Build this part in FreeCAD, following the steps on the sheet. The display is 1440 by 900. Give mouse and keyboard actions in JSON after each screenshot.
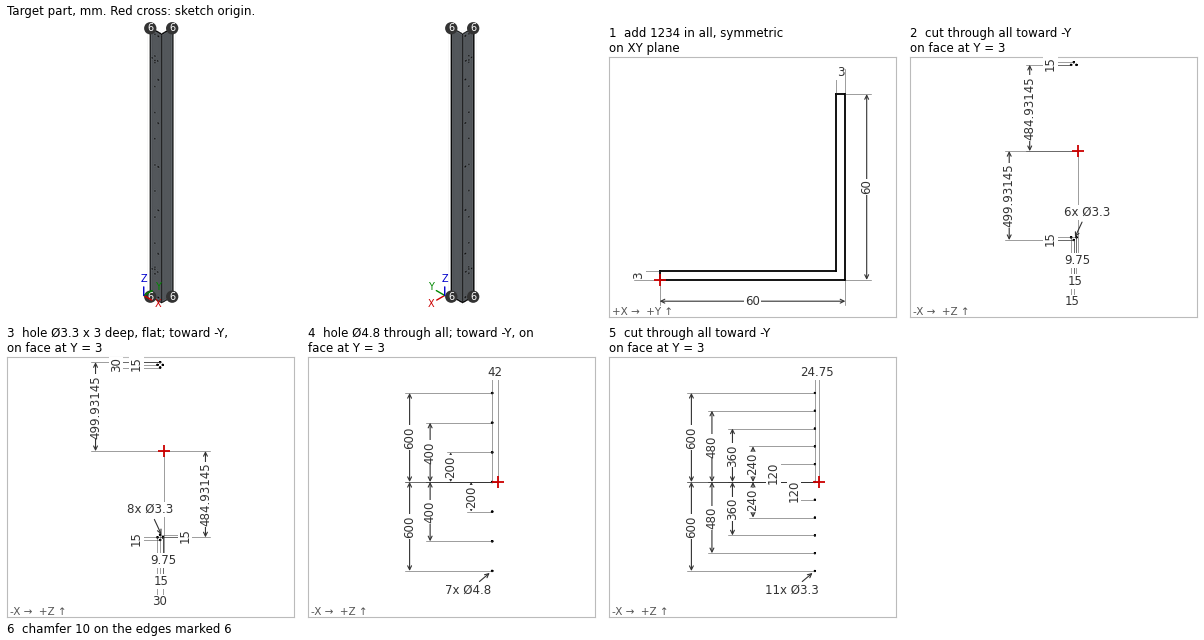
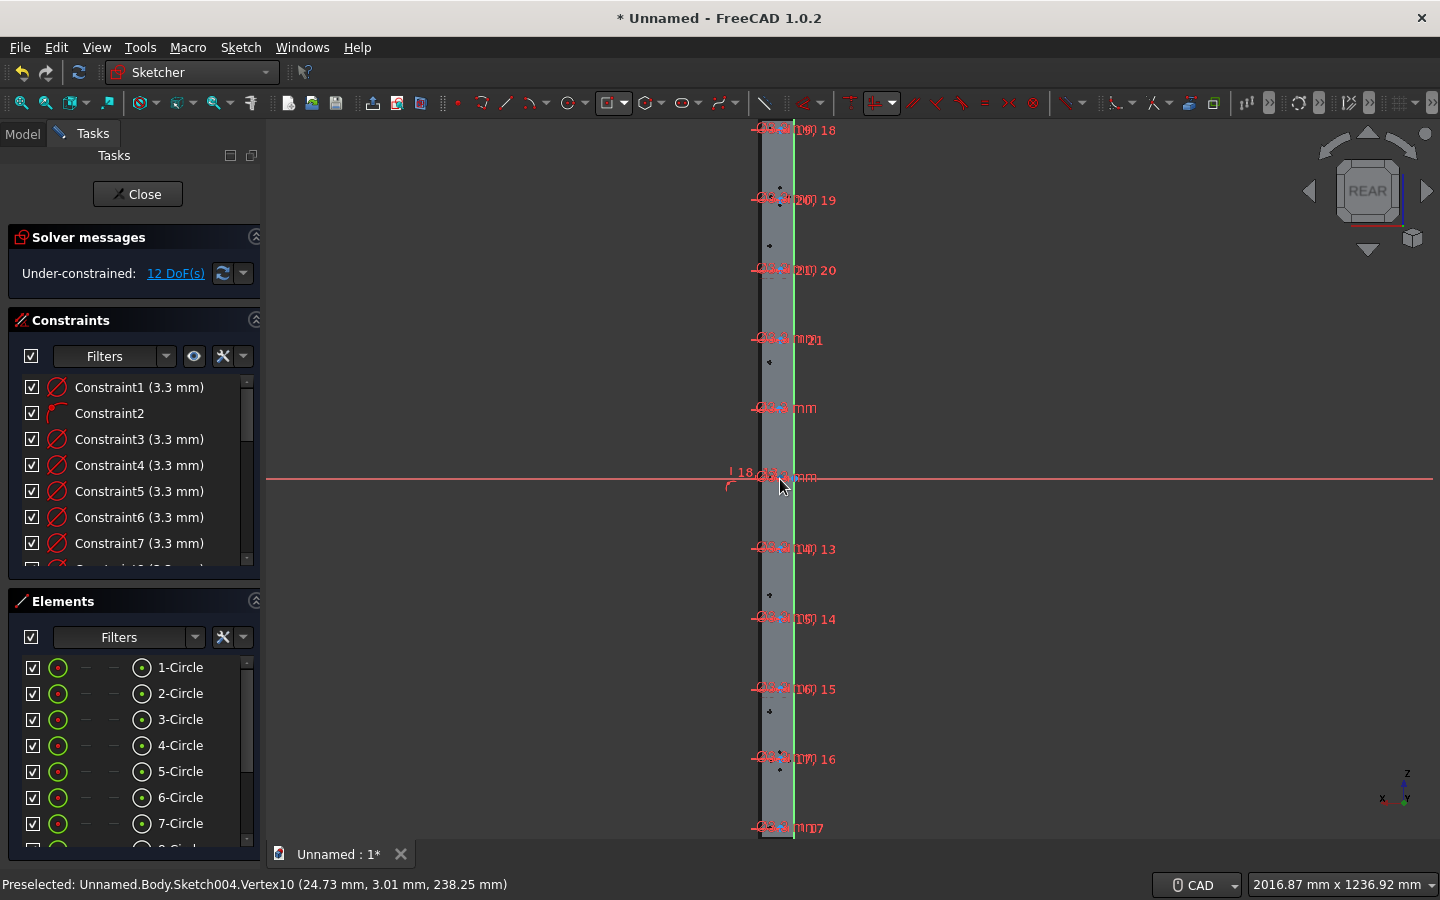
{"action": "left_click", "coordinate": [780, 479]}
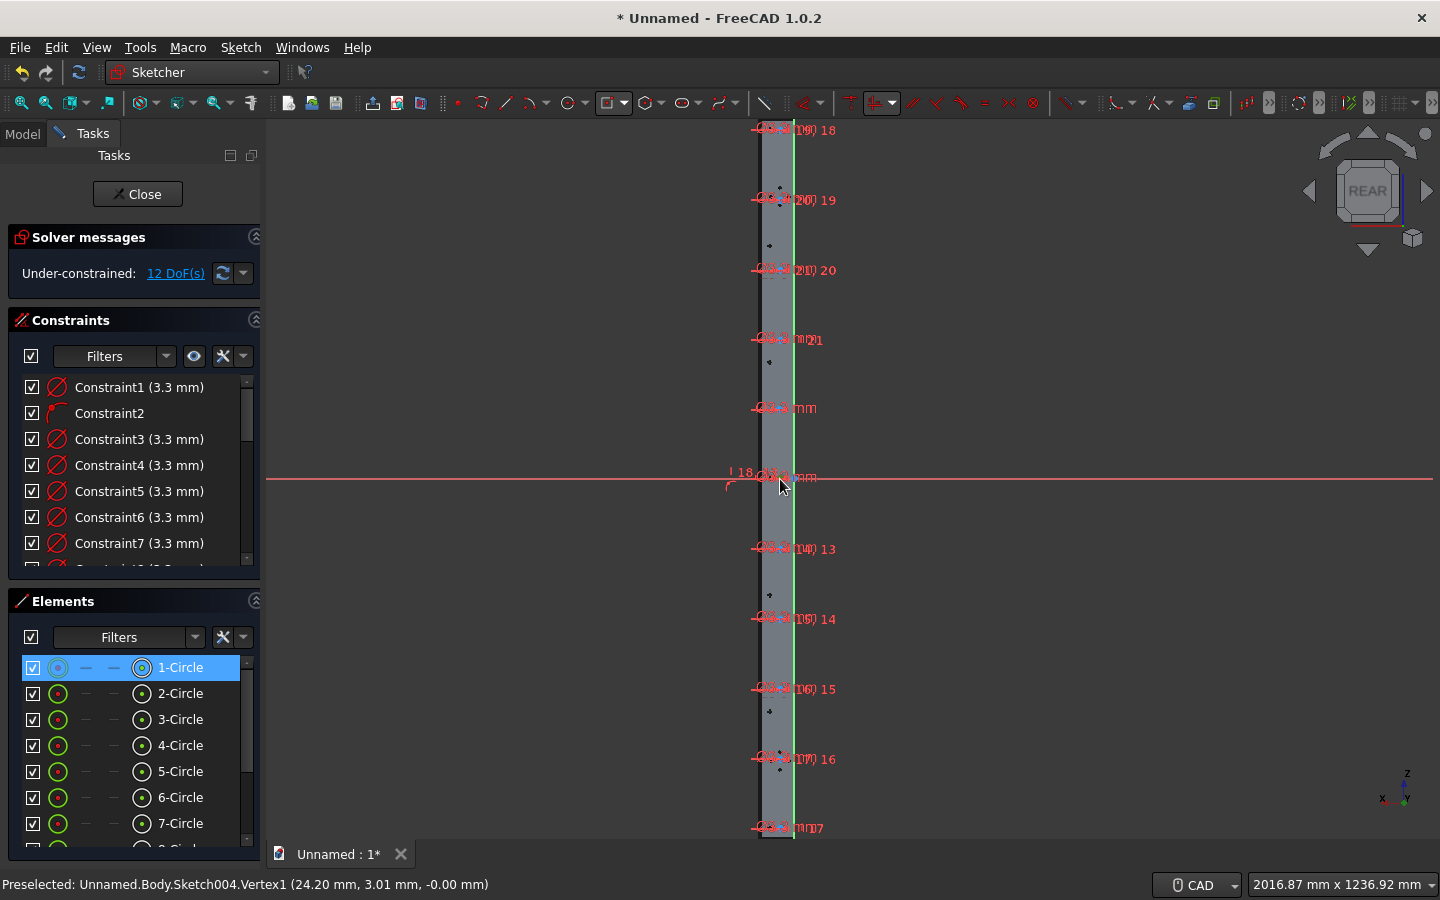
{"action": "left_click", "coordinate": [780, 410]}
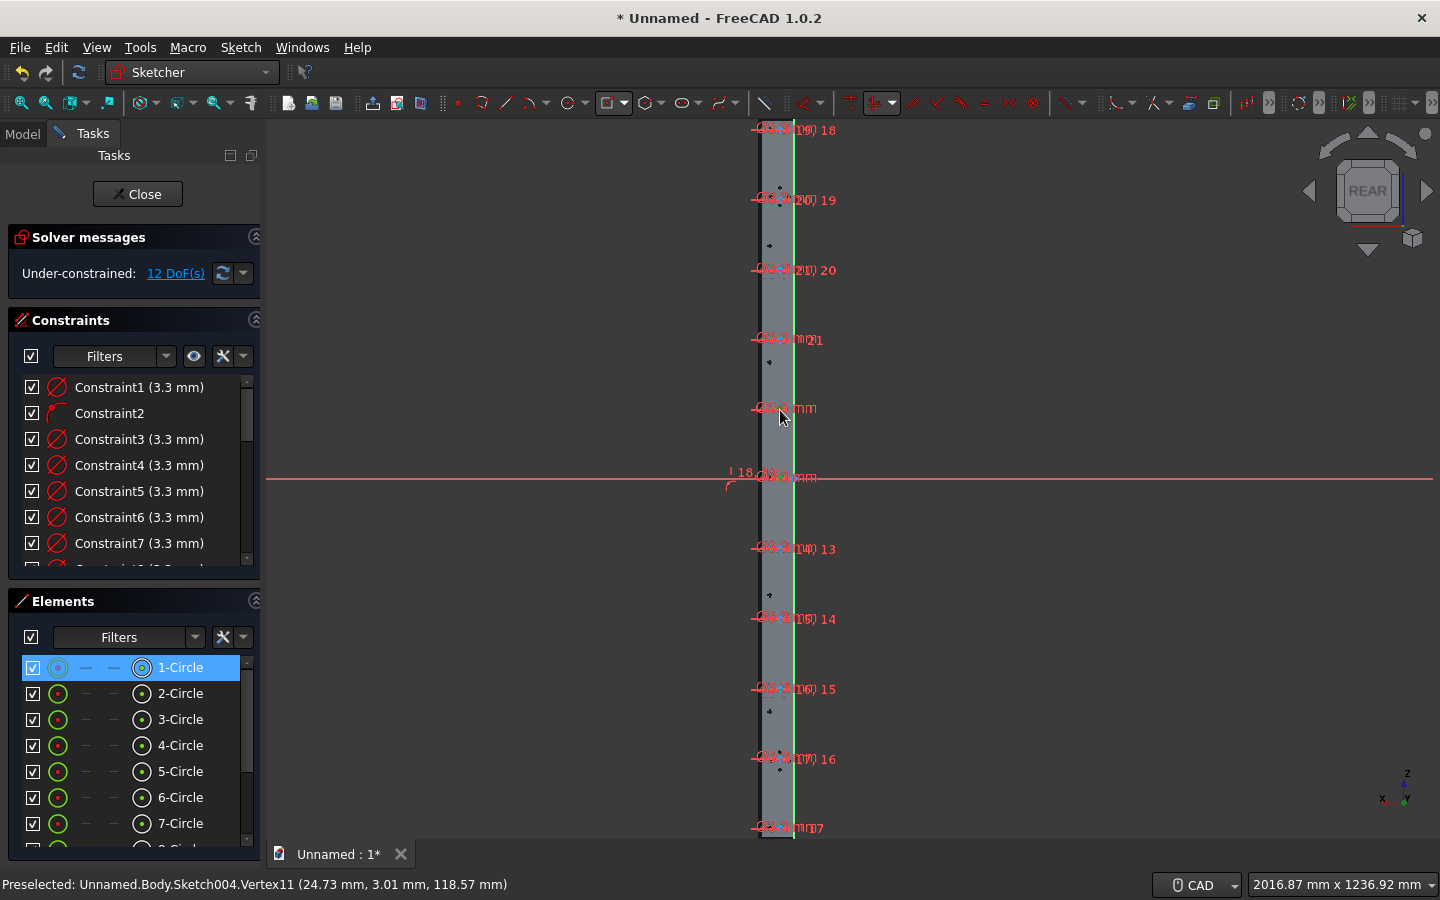
{"action": "key", "text": "v"}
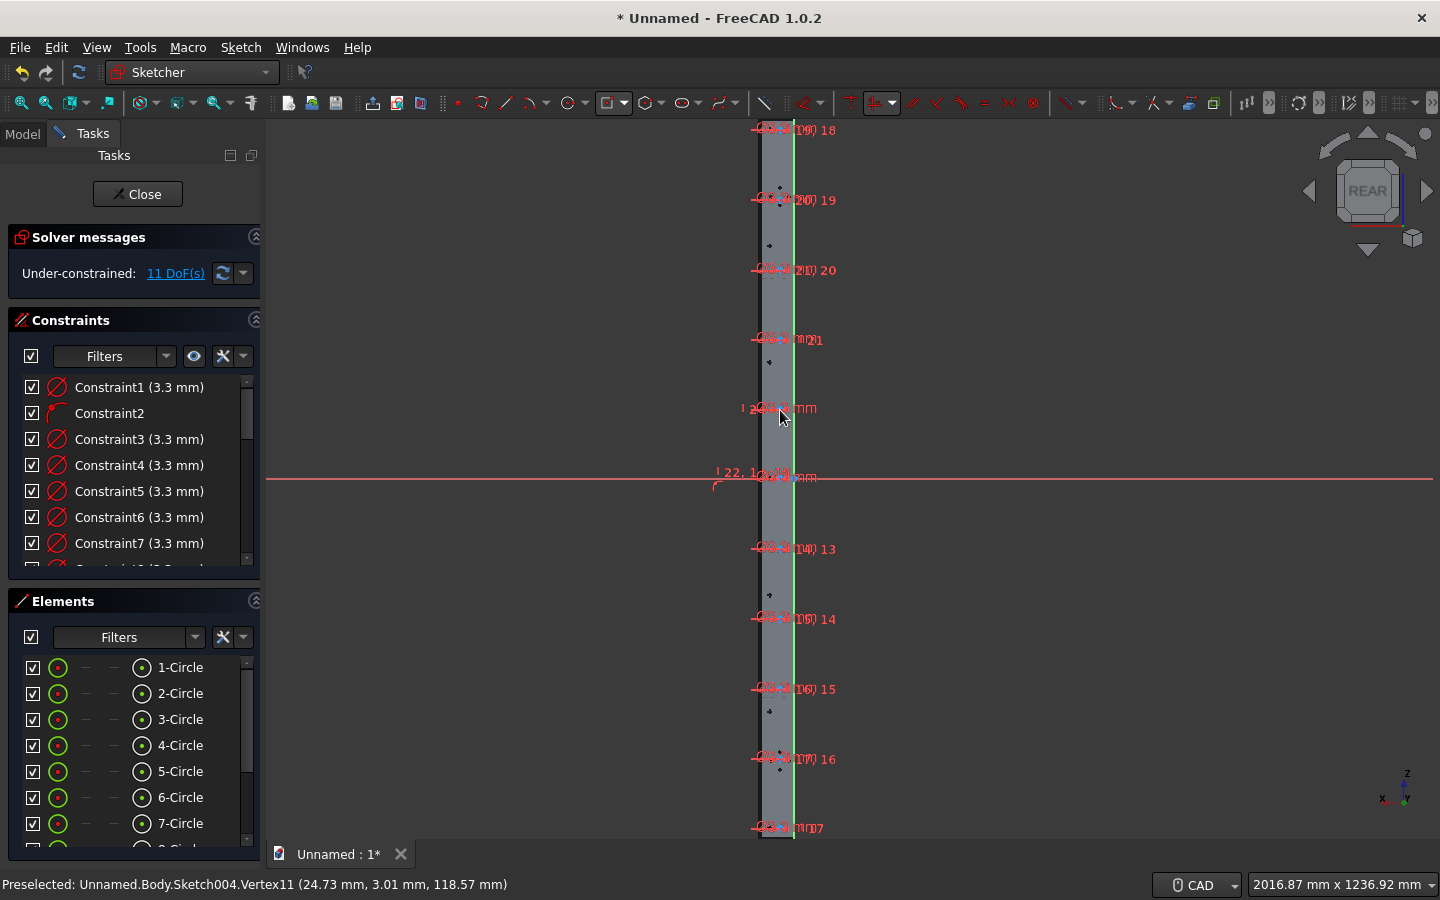
{"action": "left_click", "coordinate": [804, 104]}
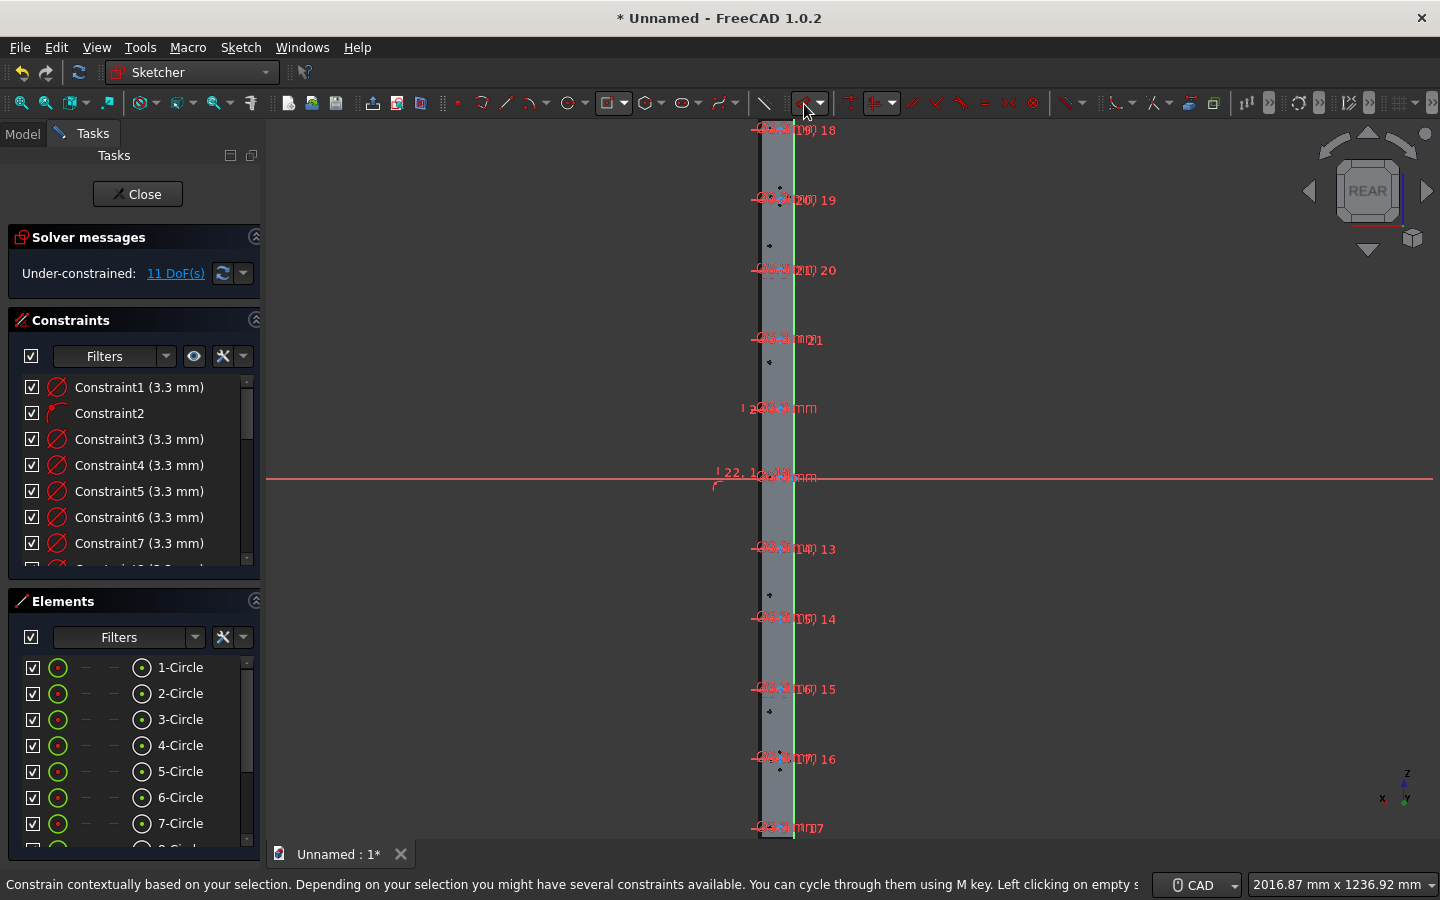
{"action": "left_click", "coordinate": [780, 549]}
{"action": "left_click", "coordinate": [828, 514]}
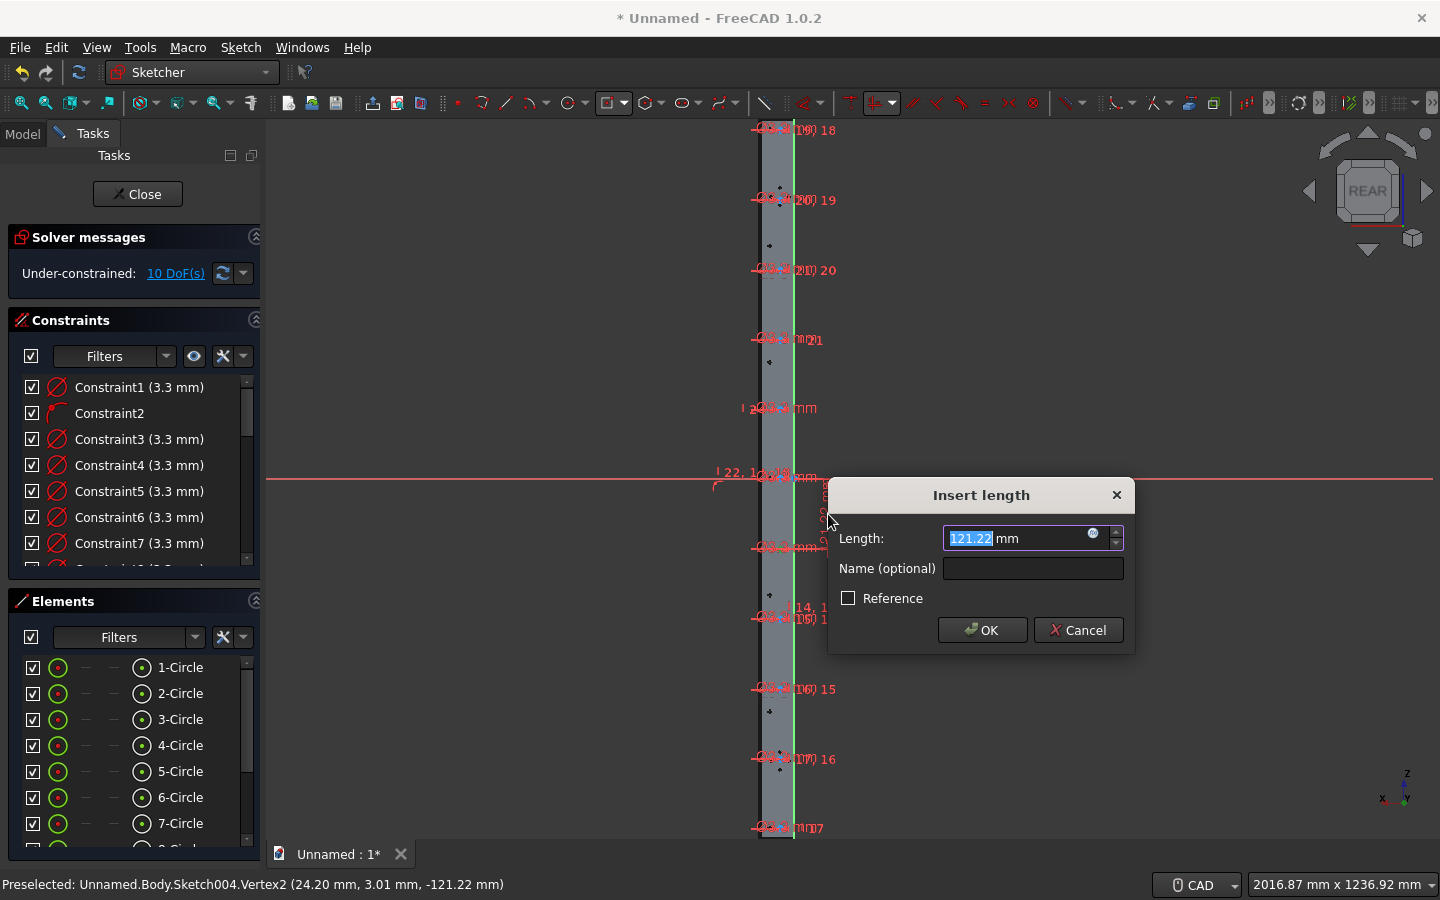
{"action": "type", "text": "120"}
{"action": "key", "text": "Return"}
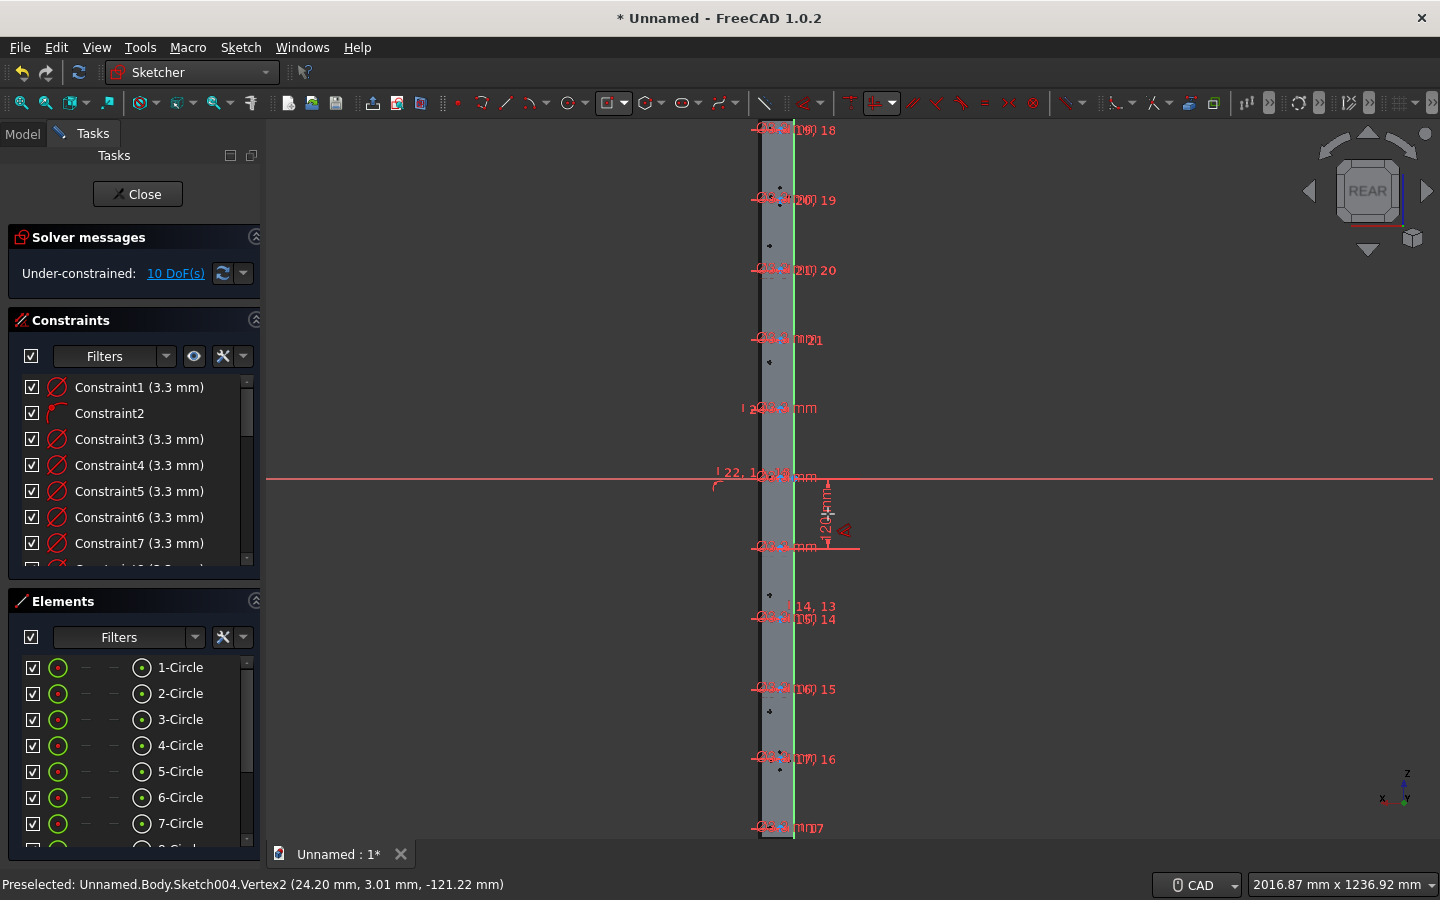
{"action": "left_click", "coordinate": [780, 619]}
{"action": "left_click", "coordinate": [828, 549]}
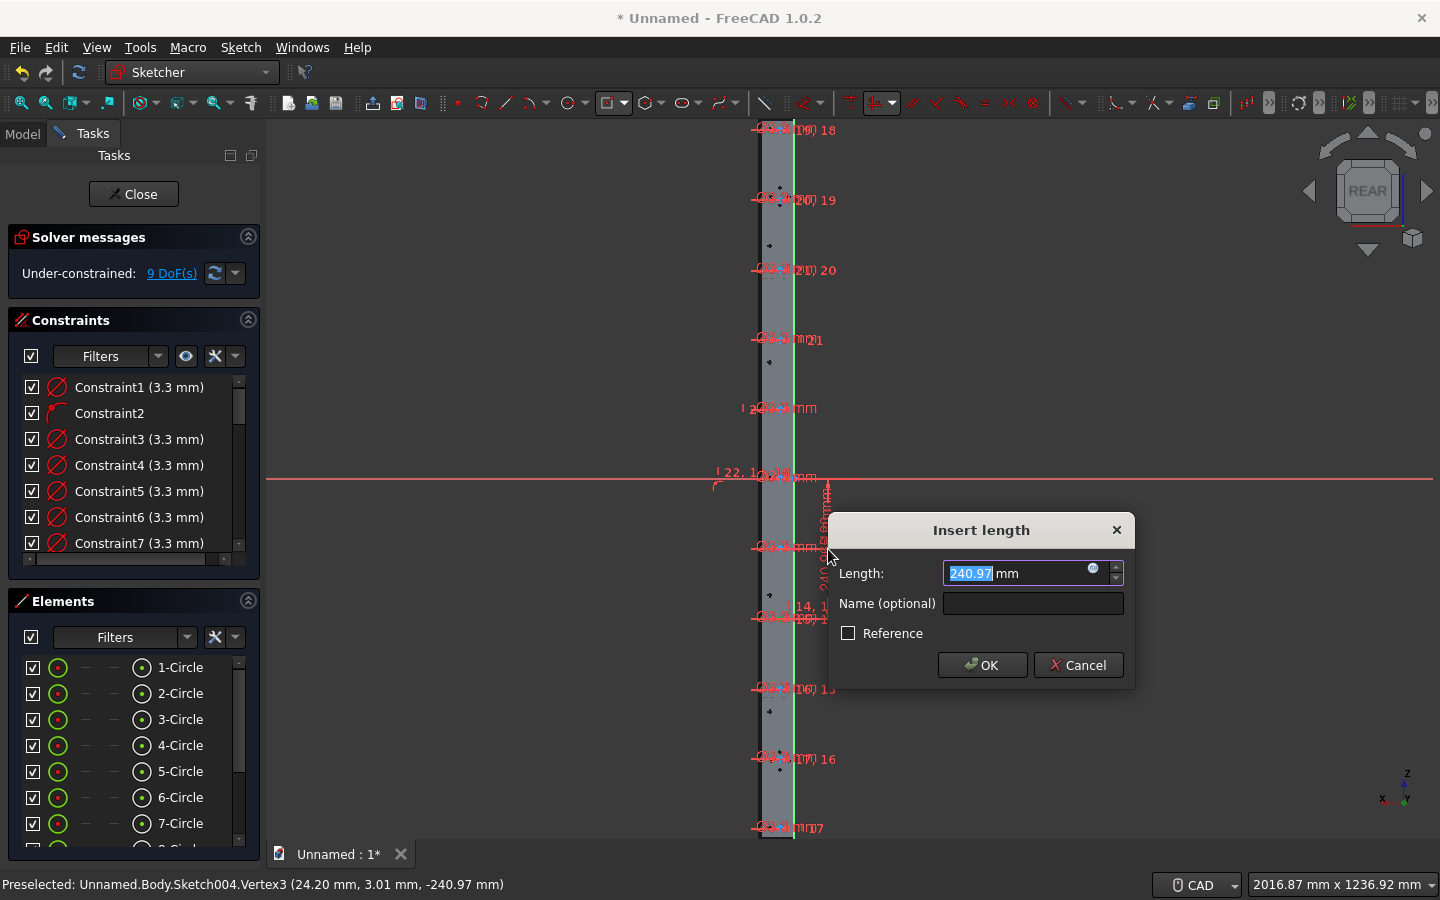
{"action": "type", "text": "240"}
{"action": "key", "text": "Return"}